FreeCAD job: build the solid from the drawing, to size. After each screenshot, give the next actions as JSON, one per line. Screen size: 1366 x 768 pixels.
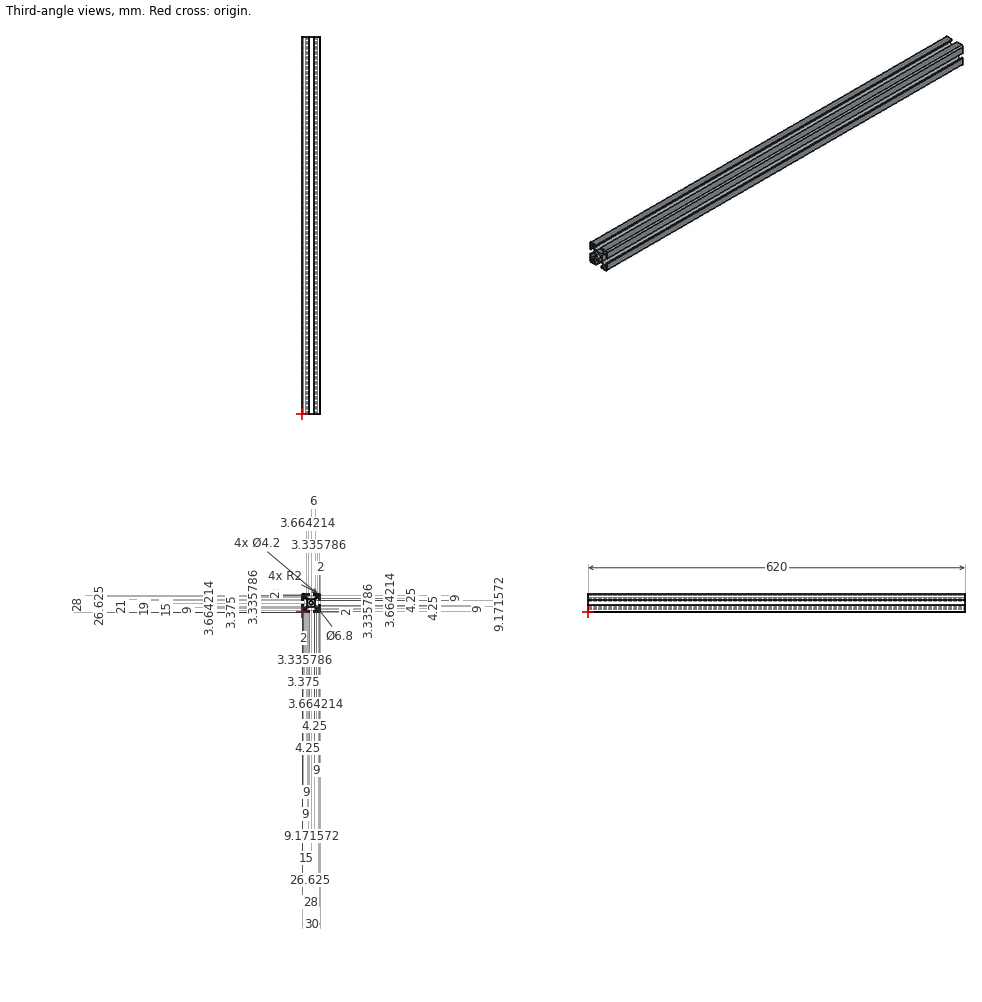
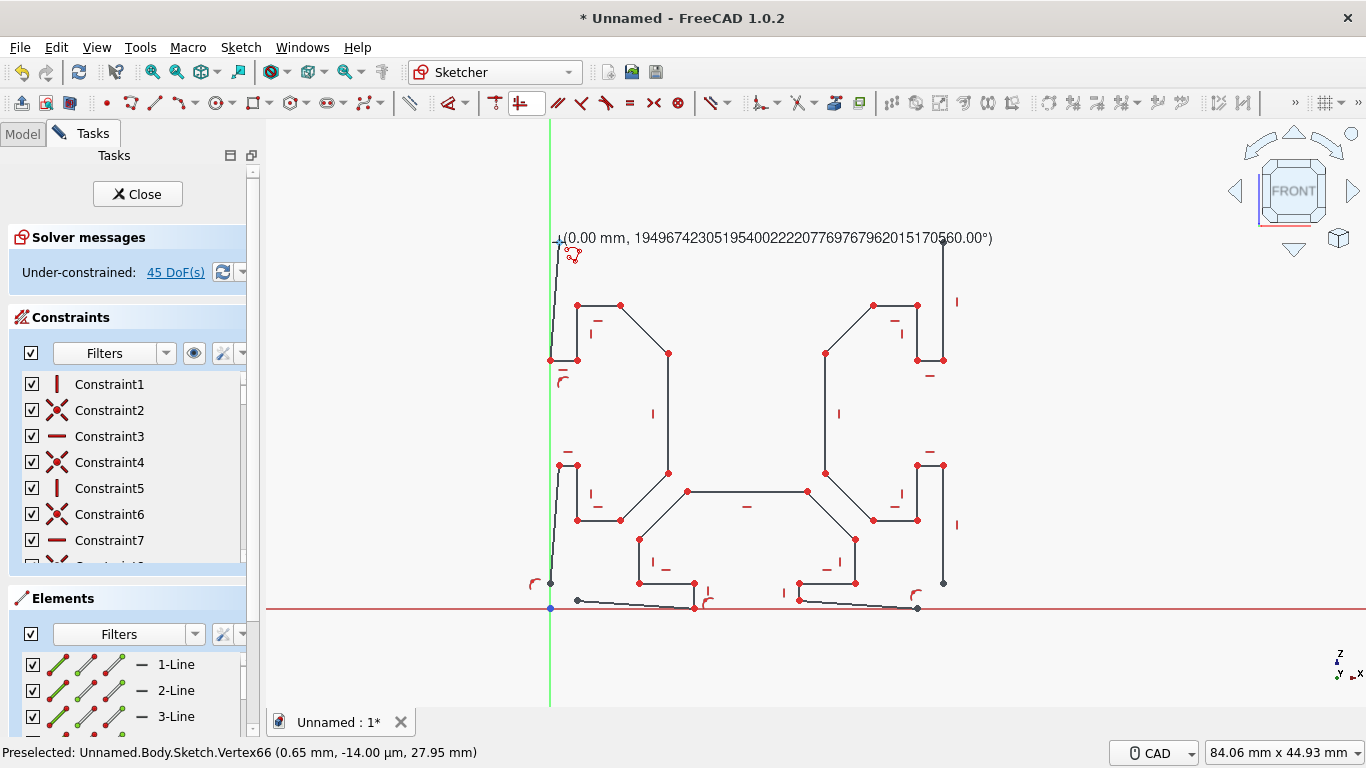
{"action": "left_click", "coordinate": [577, 216]}
{"action": "left_click", "coordinate": [694, 216]}
{"action": "left_click", "coordinate": [694, 242]}
{"action": "left_click", "coordinate": [639, 242]}
{"action": "left_click", "coordinate": [639, 286]}
{"action": "left_click", "coordinate": [687, 334]}
{"action": "left_click", "coordinate": [807, 334]}
{"action": "left_click", "coordinate": [855, 286]}
{"action": "left_click", "coordinate": [855, 242]}
{"action": "left_click", "coordinate": [799, 242]}
{"action": "left_click", "coordinate": [799, 216]}
{"action": "left_click", "coordinate": [917, 216]}
{"action": "right_click", "coordinate": [917, 216]}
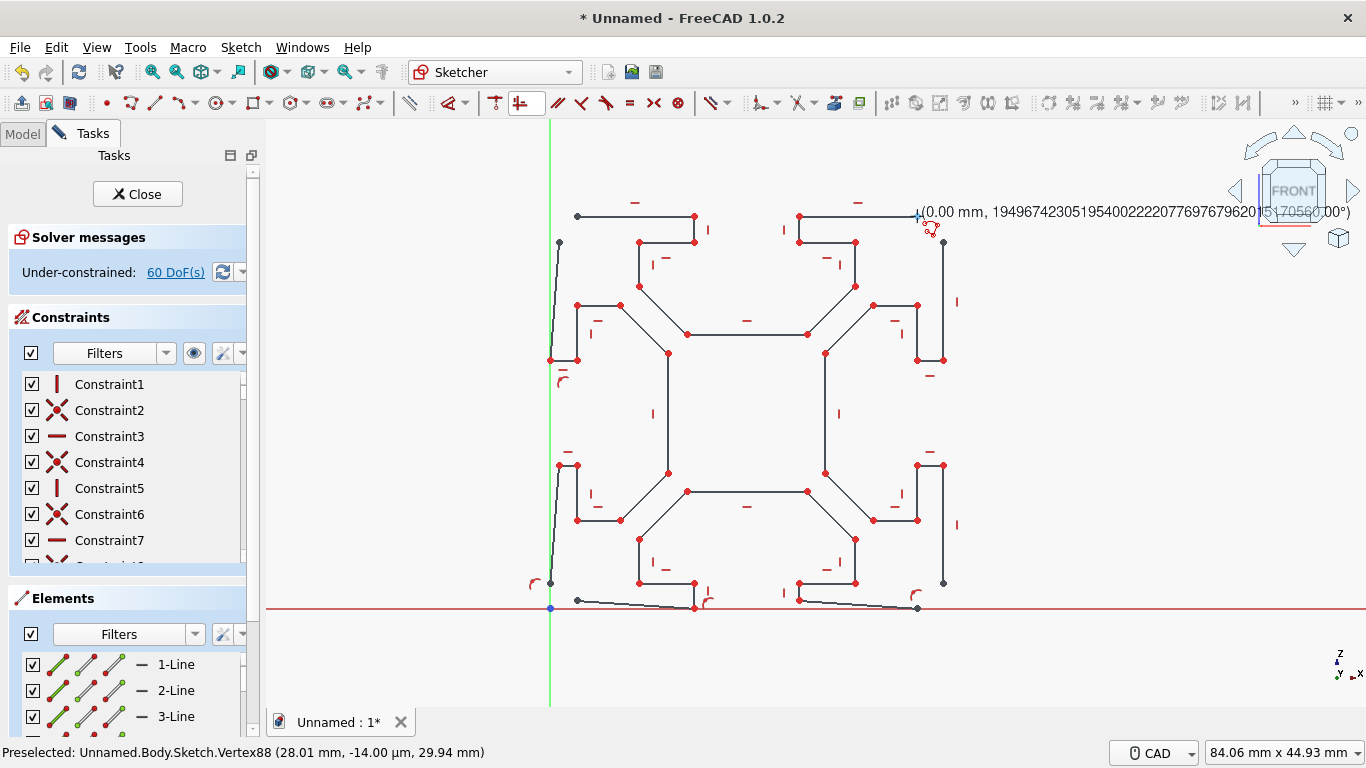
{"action": "key", "text": "g 3 a"}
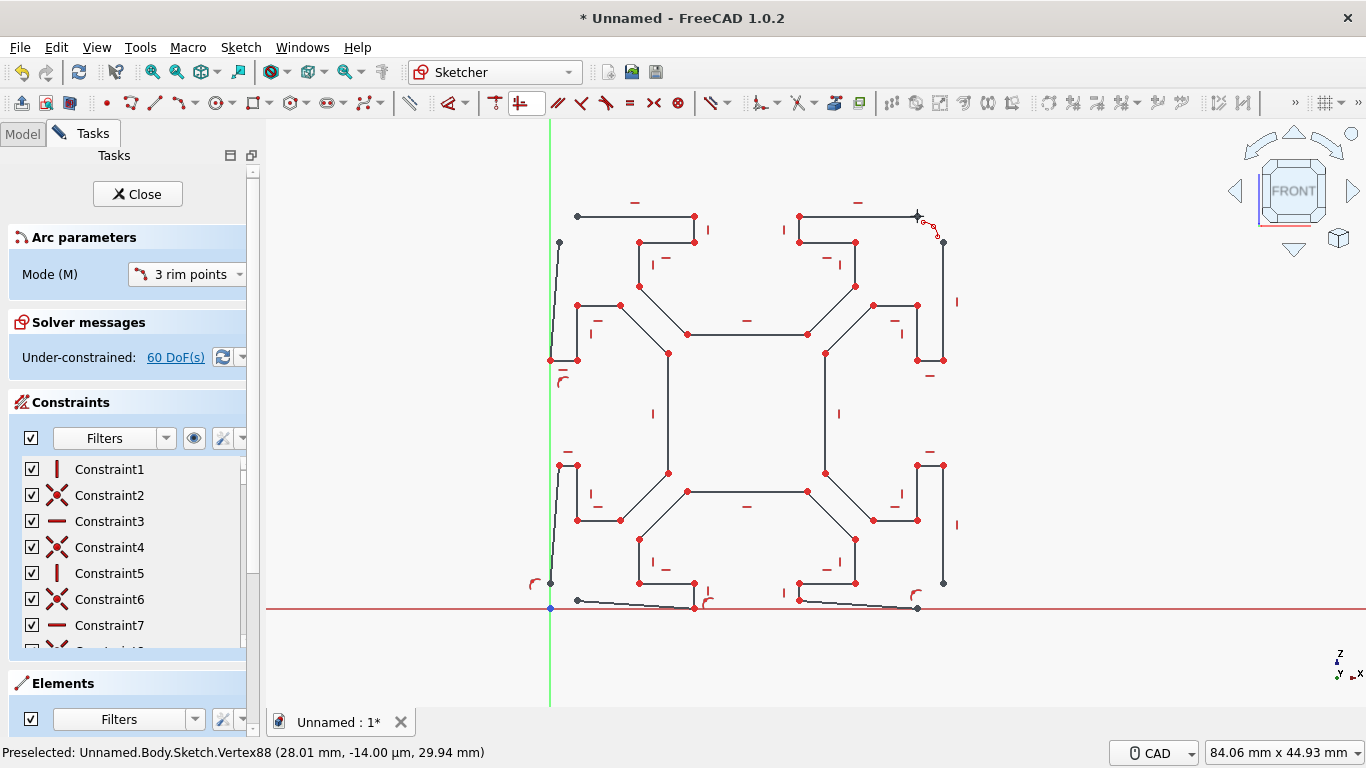
{"action": "left_click", "coordinate": [943, 584]}
{"action": "left_click", "coordinate": [917, 609]}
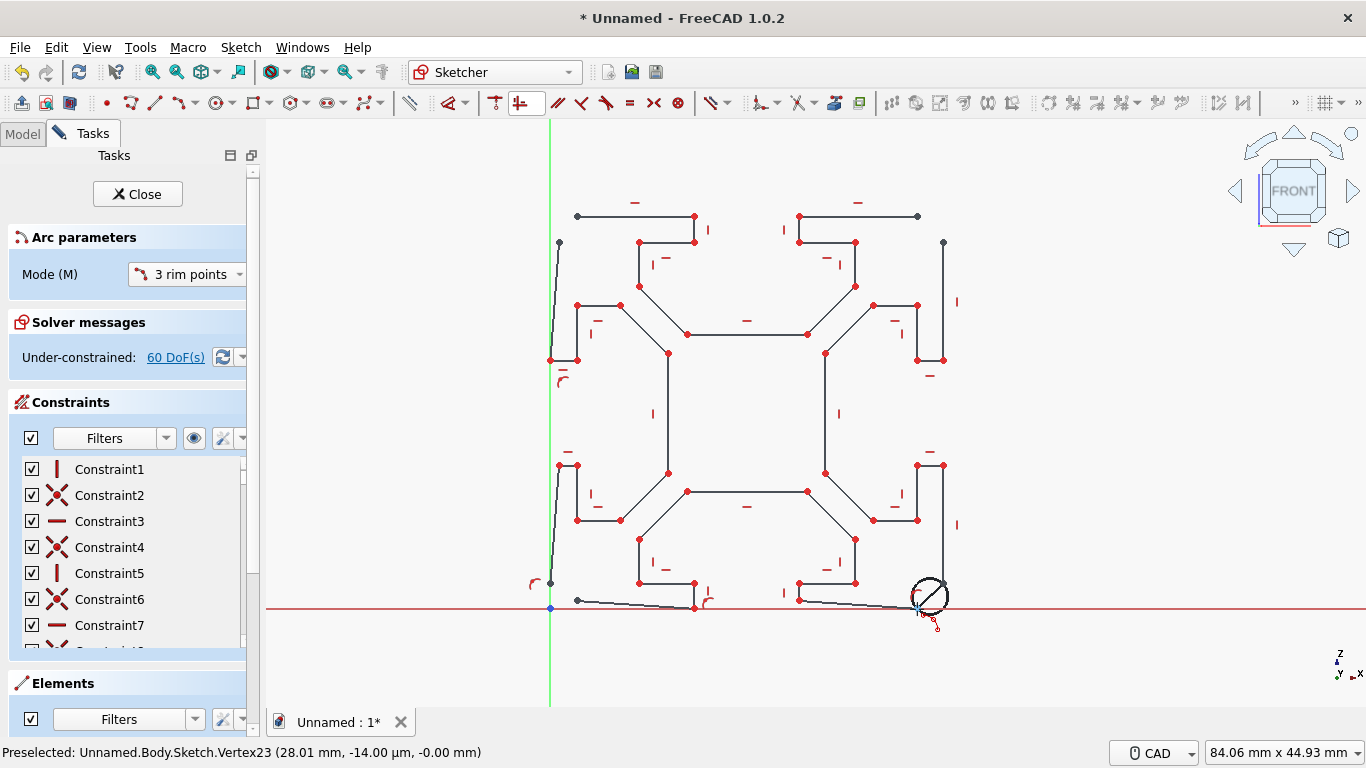
{"action": "scroll", "coordinate": [935, 601], "scroll_direction": "up", "scroll_amount": 4}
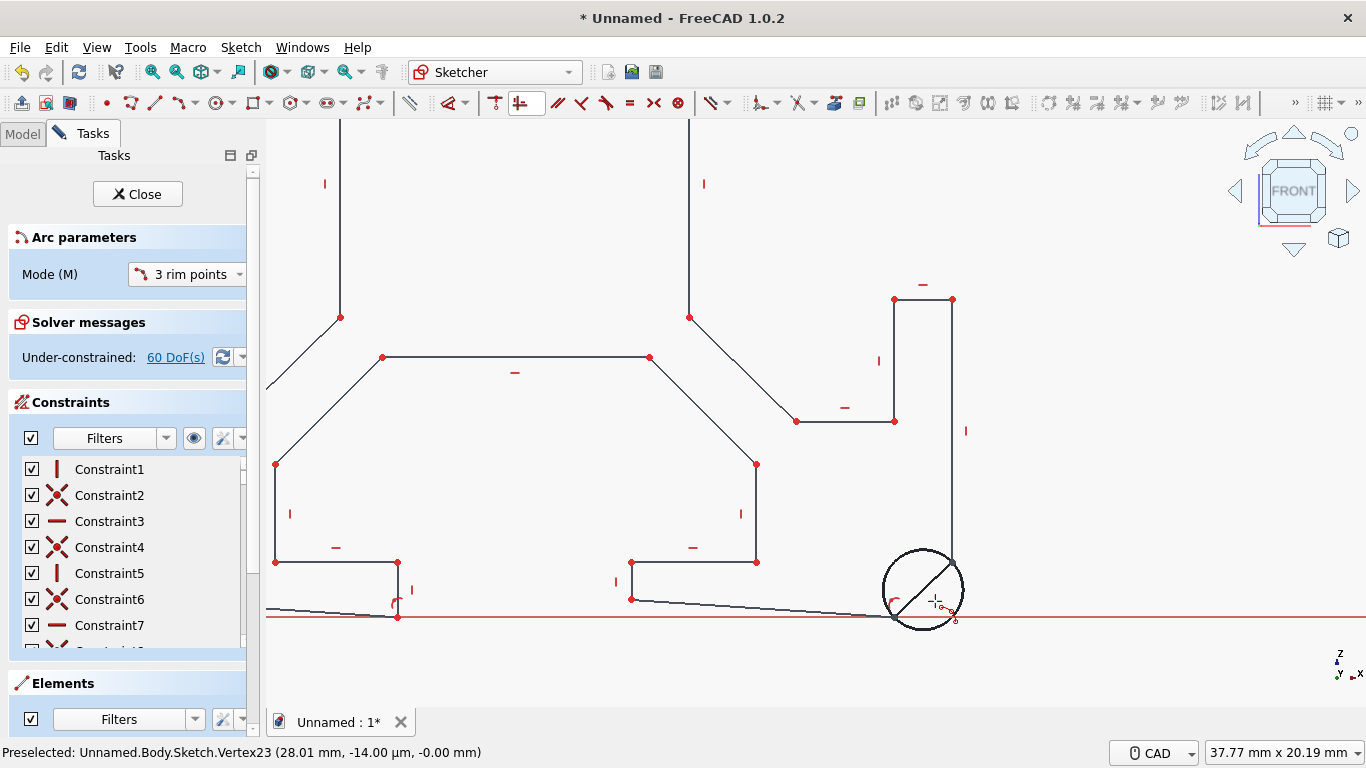
{"action": "left_click", "coordinate": [935, 600]}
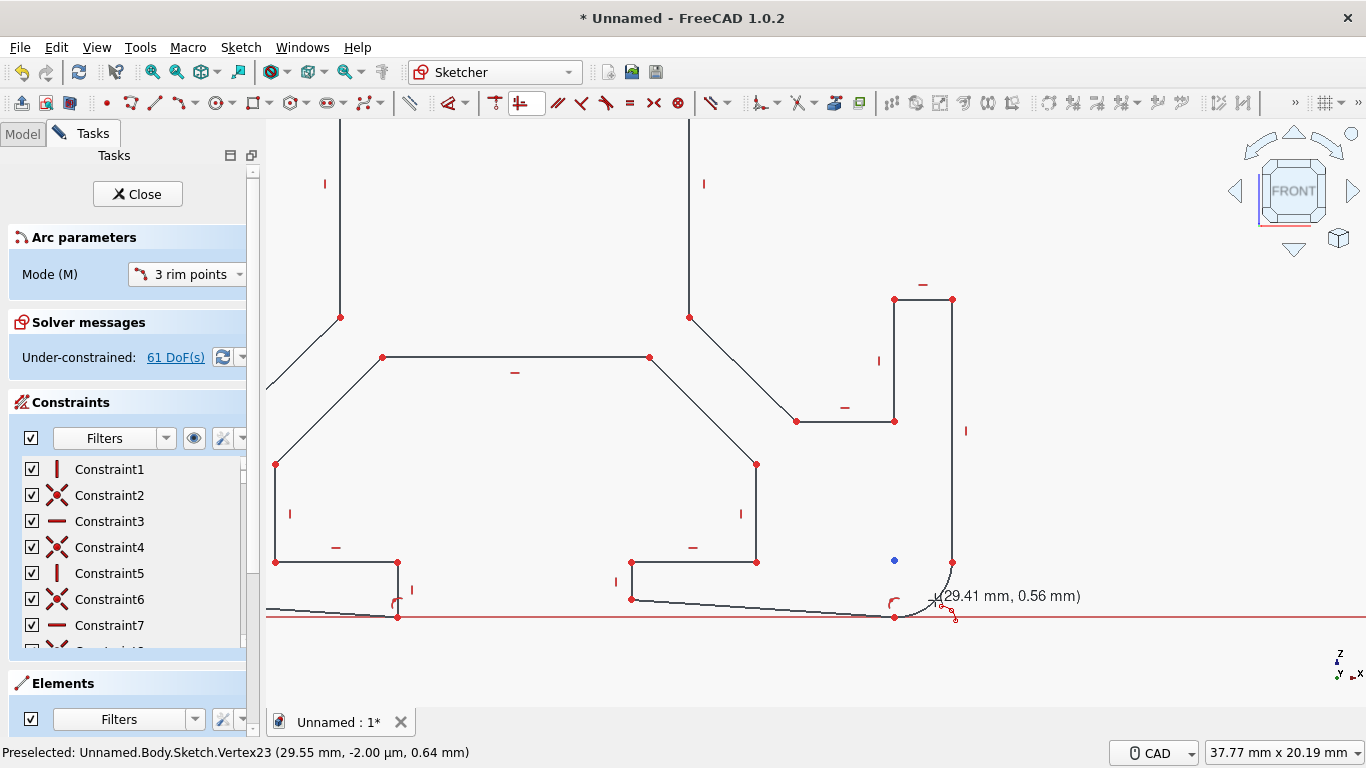
{"action": "scroll", "coordinate": [937, 603], "scroll_direction": "down", "scroll_amount": 4}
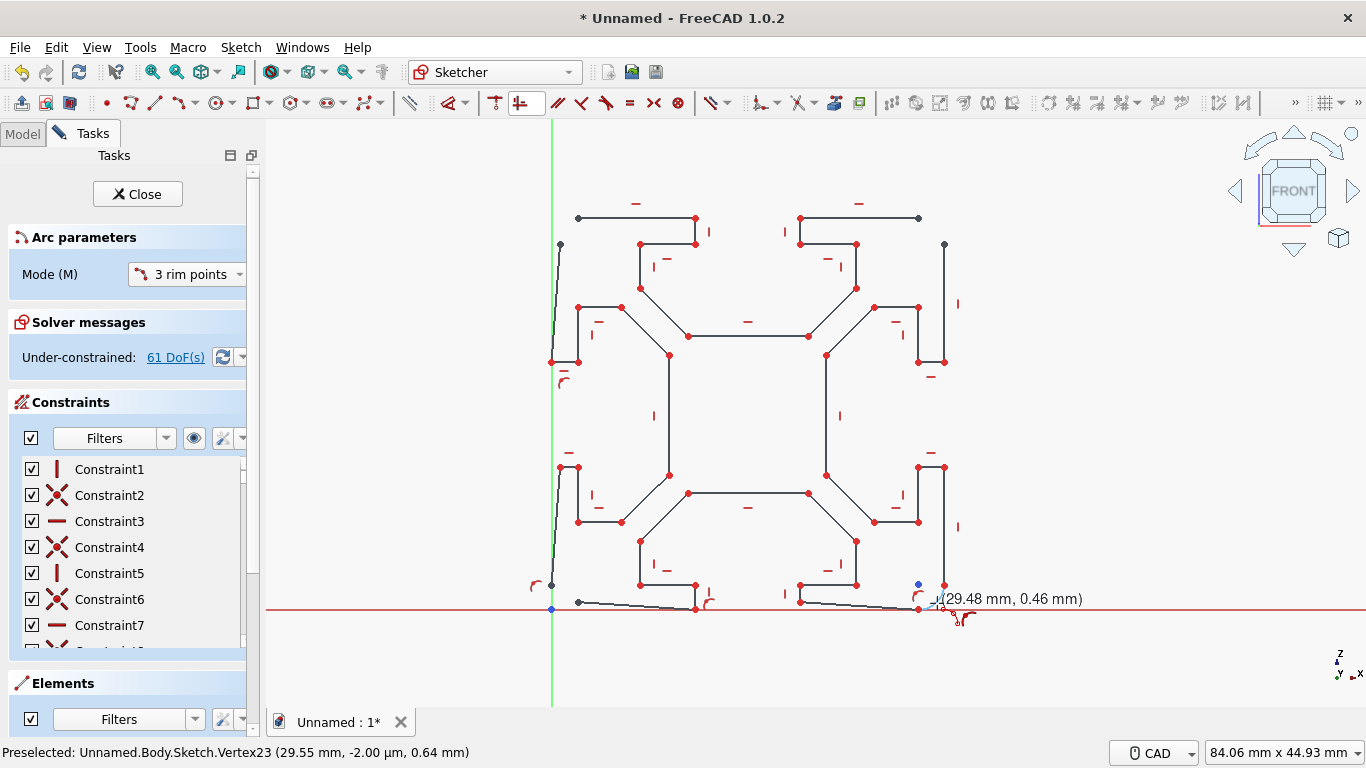
{"action": "left_click", "coordinate": [578, 602]}
{"action": "left_click", "coordinate": [552, 585]}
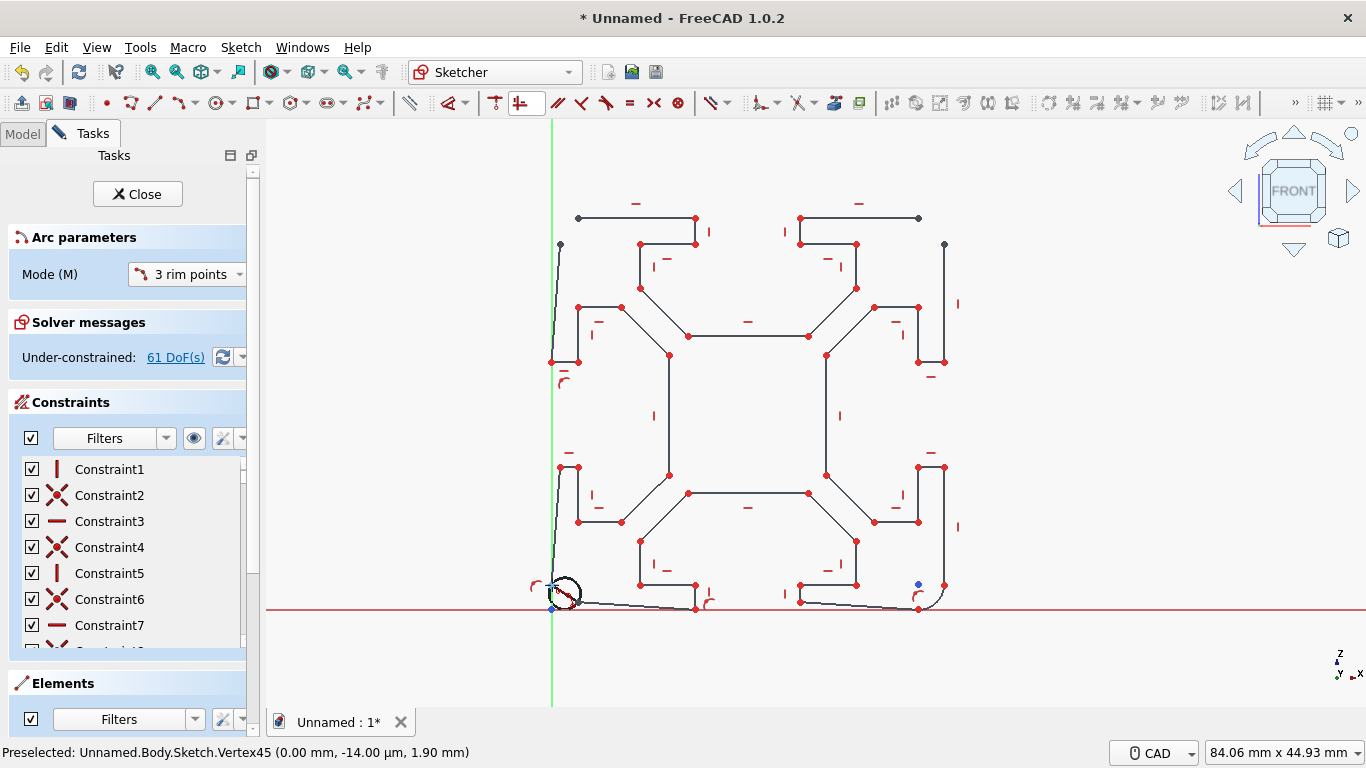
{"action": "scroll", "coordinate": [559, 602], "scroll_direction": "up", "scroll_amount": 4}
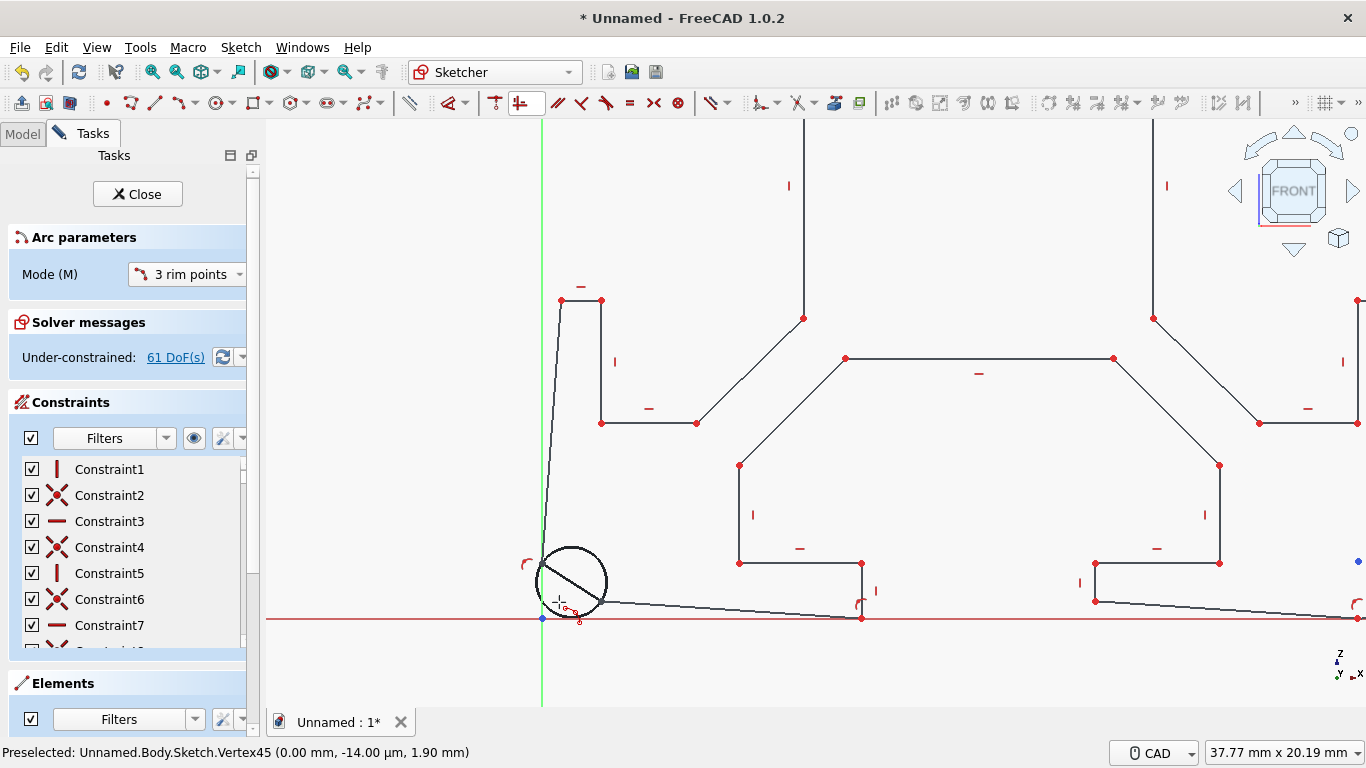
{"action": "left_click", "coordinate": [559, 602]}